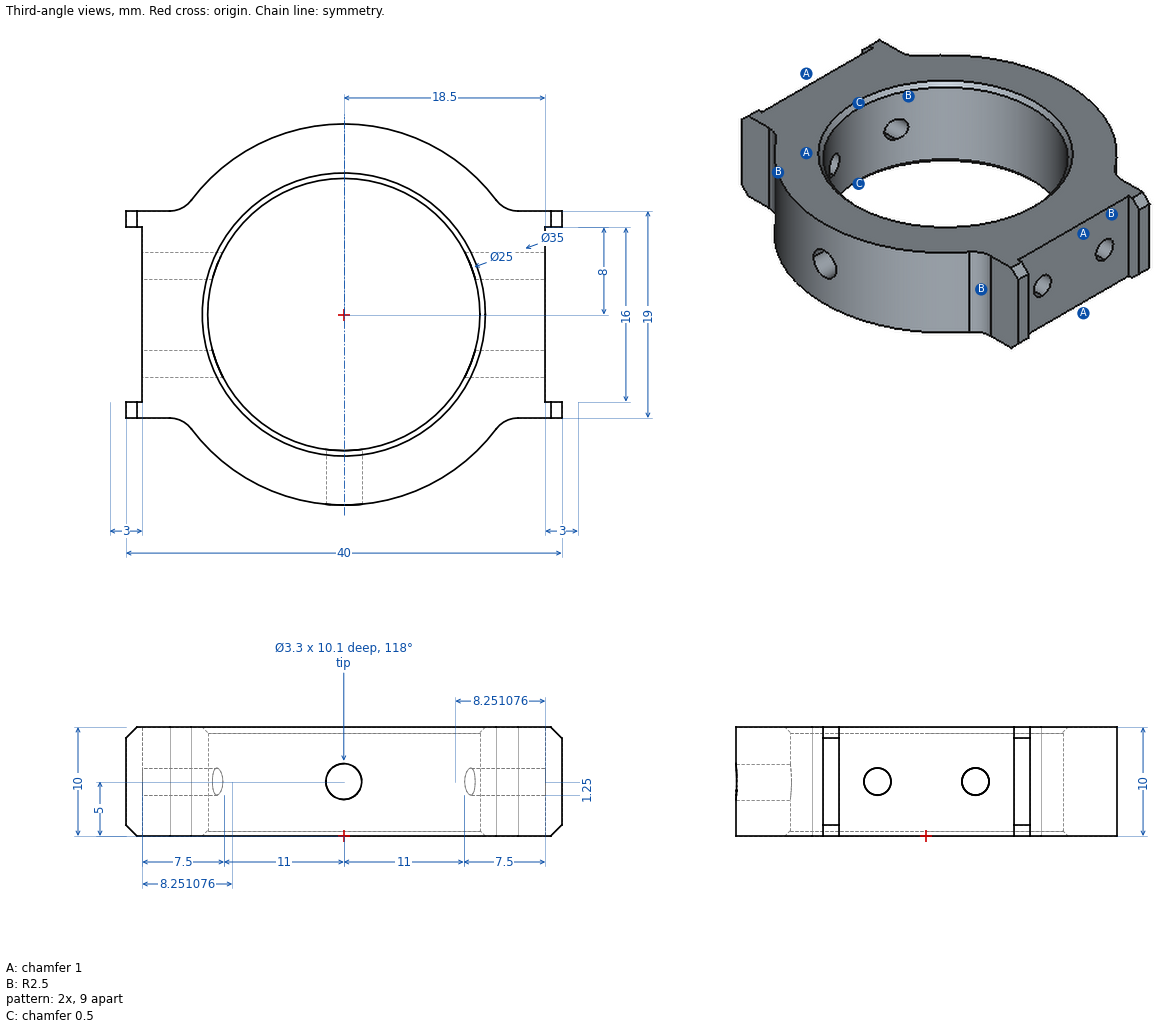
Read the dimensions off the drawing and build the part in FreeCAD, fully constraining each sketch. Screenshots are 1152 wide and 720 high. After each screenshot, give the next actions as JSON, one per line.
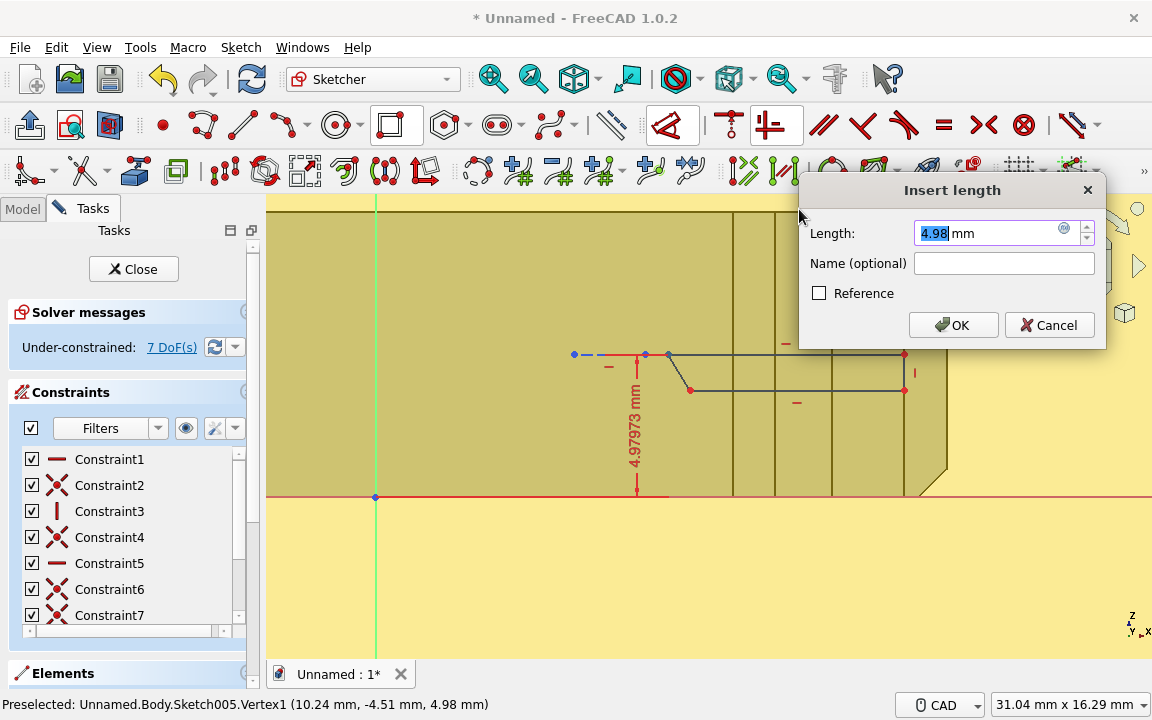
{"action": "type", "text": "5"}
{"action": "key", "text": "Return"}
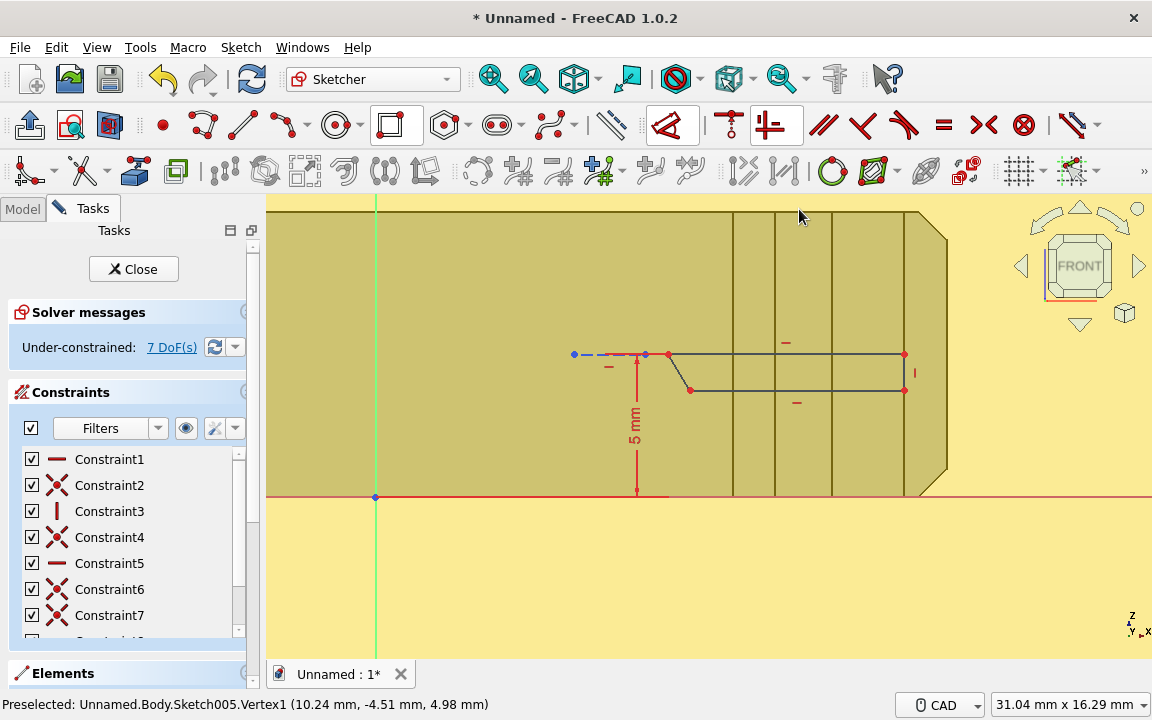
{"action": "left_click", "coordinate": [645, 355]}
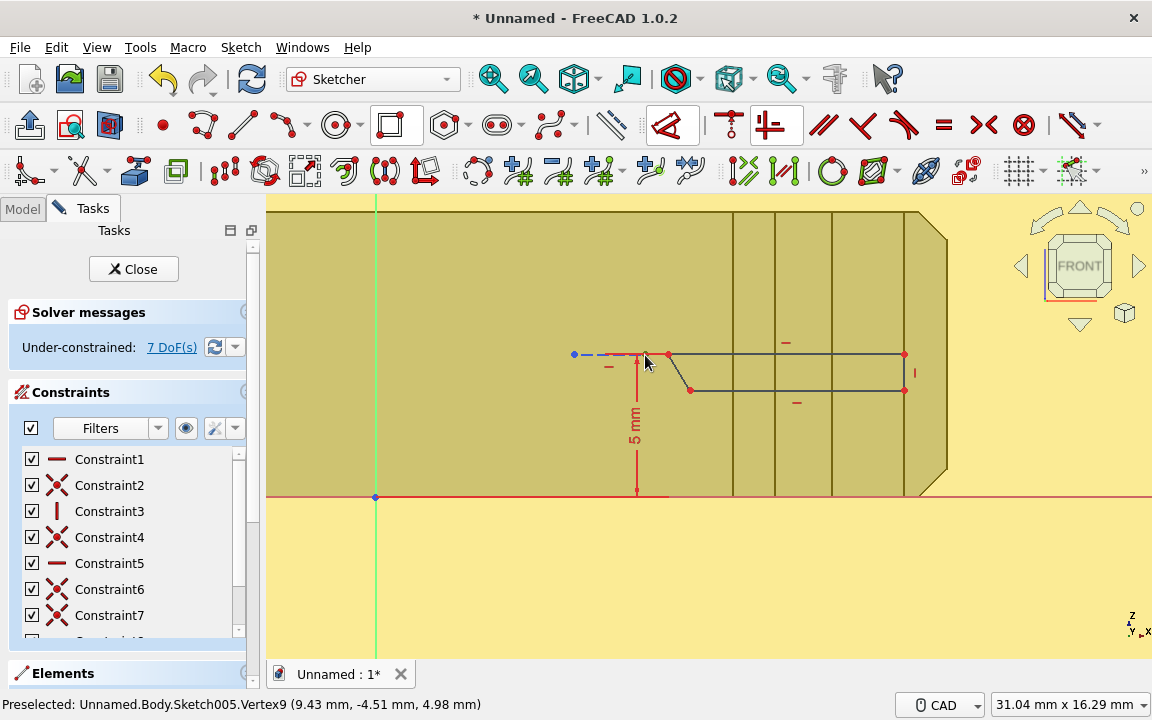
{"action": "key", "text": "i"}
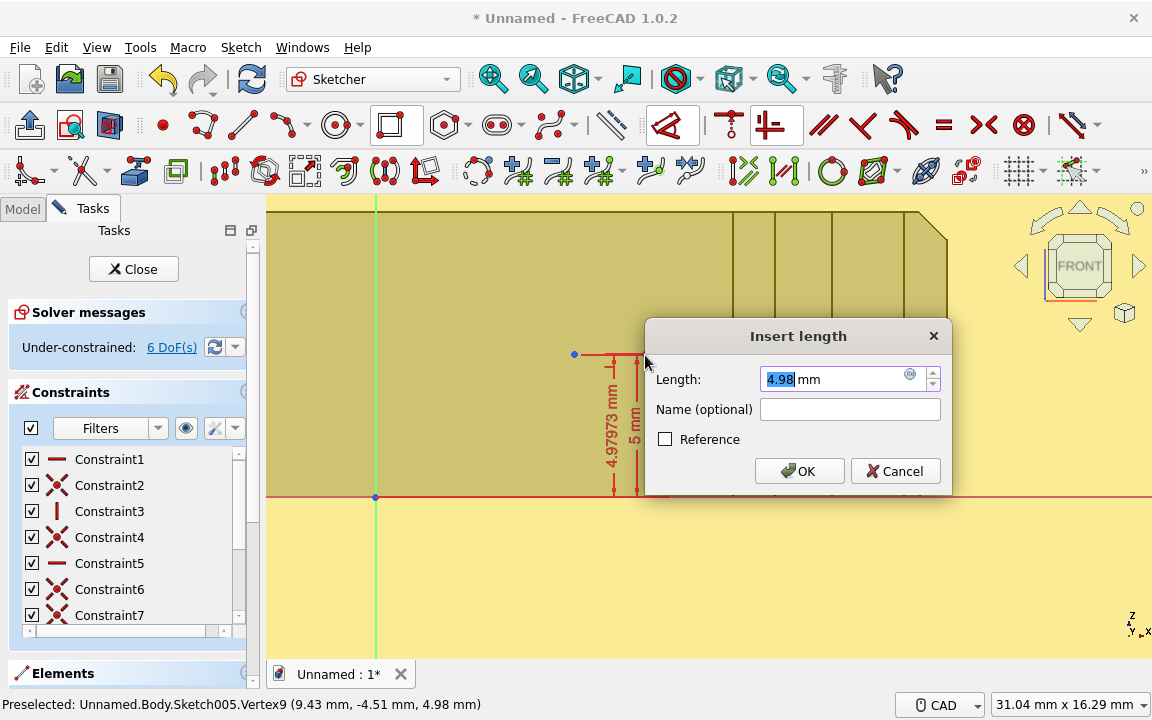
{"action": "type", "text": "5"}
{"action": "key", "text": "Return"}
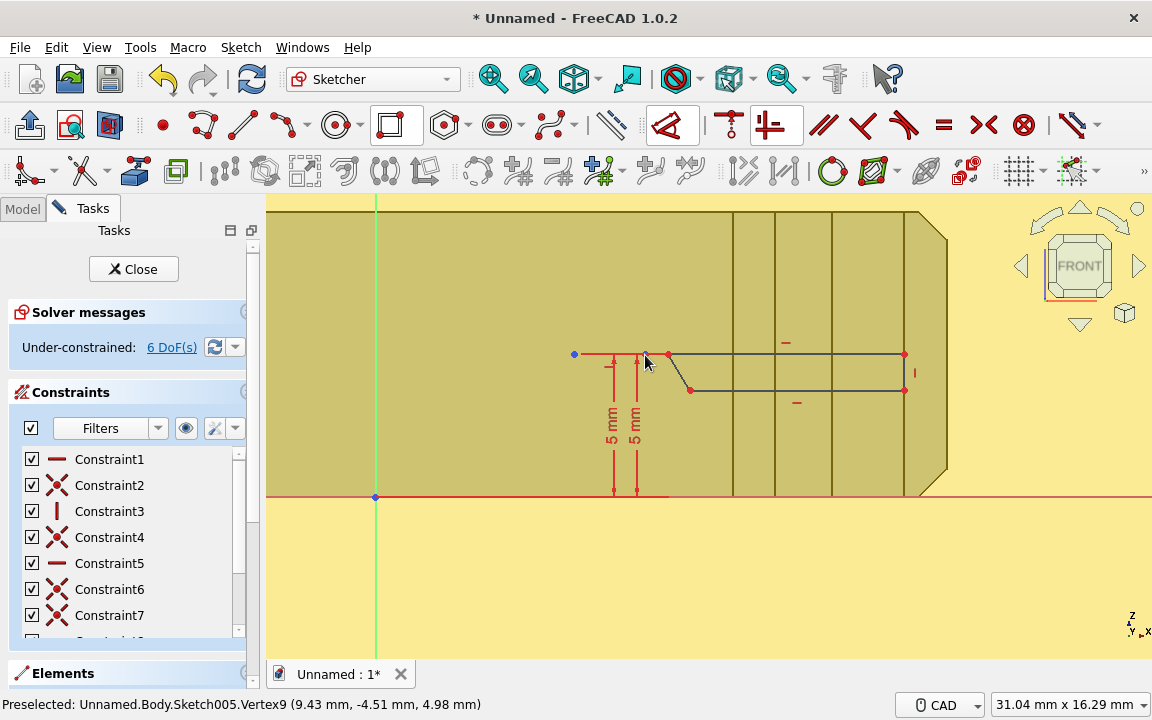
{"action": "left_click", "coordinate": [840, 391]}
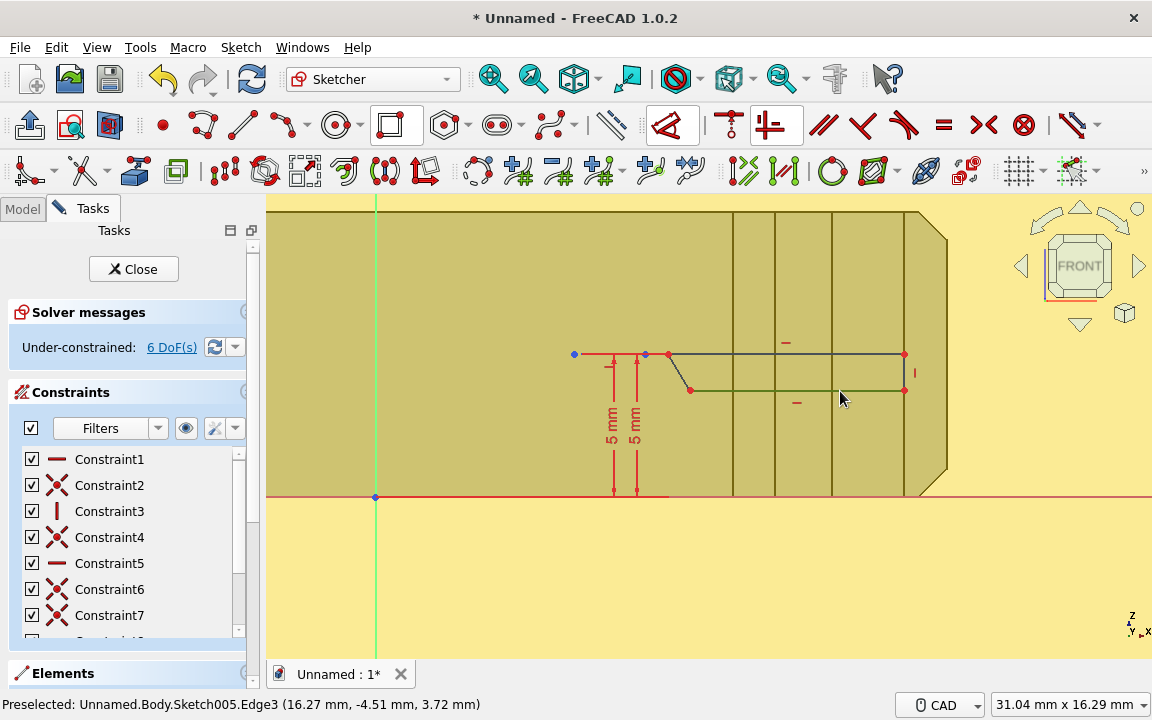
{"action": "left_click", "coordinate": [694, 126]}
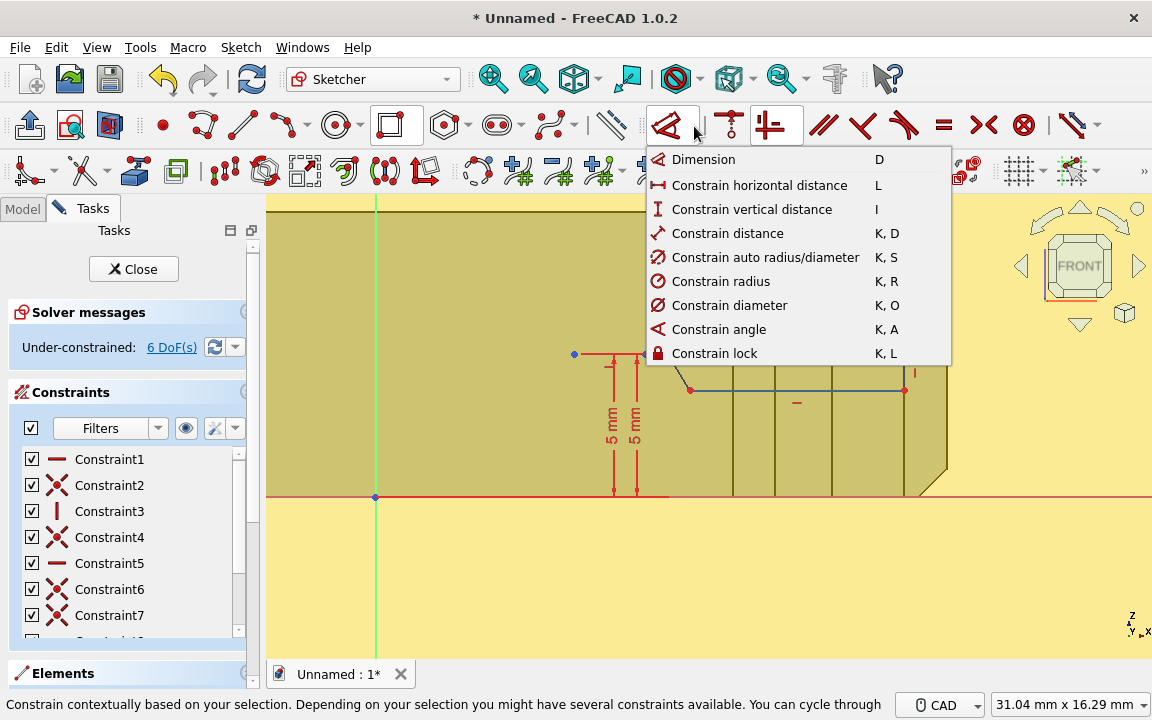
{"action": "left_click", "coordinate": [799, 185]}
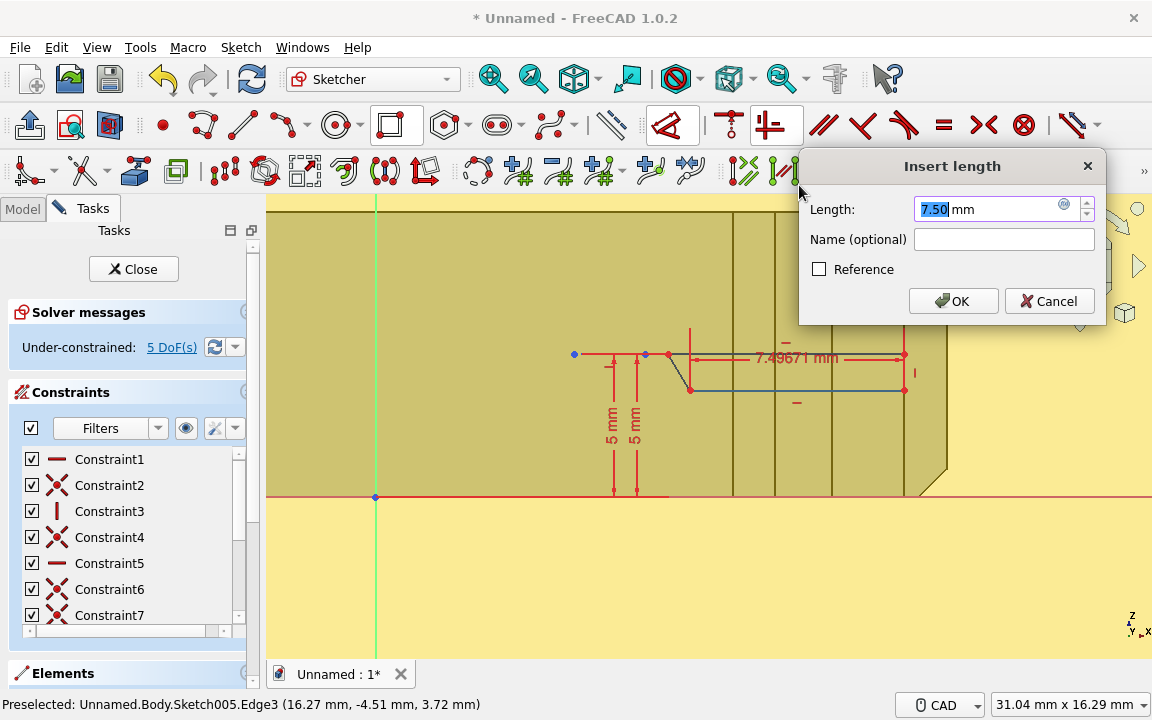
{"action": "type", "text": "7.5"}
{"action": "key", "text": "Return"}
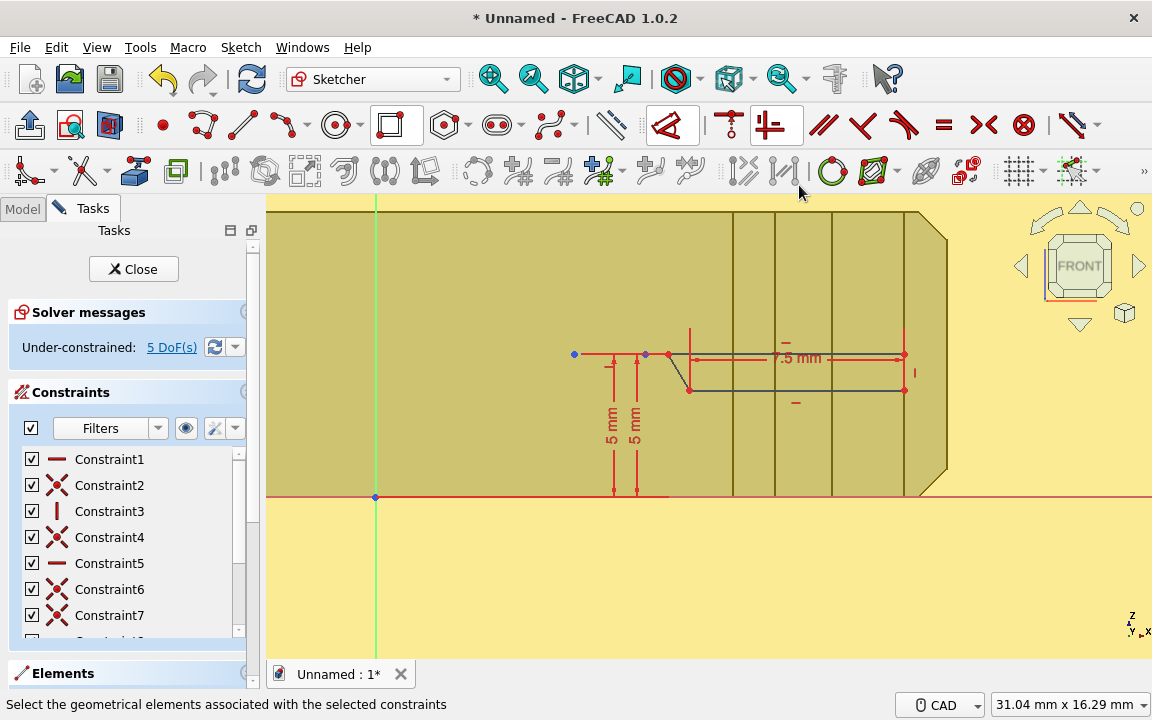
{"action": "left_click", "coordinate": [690, 391]}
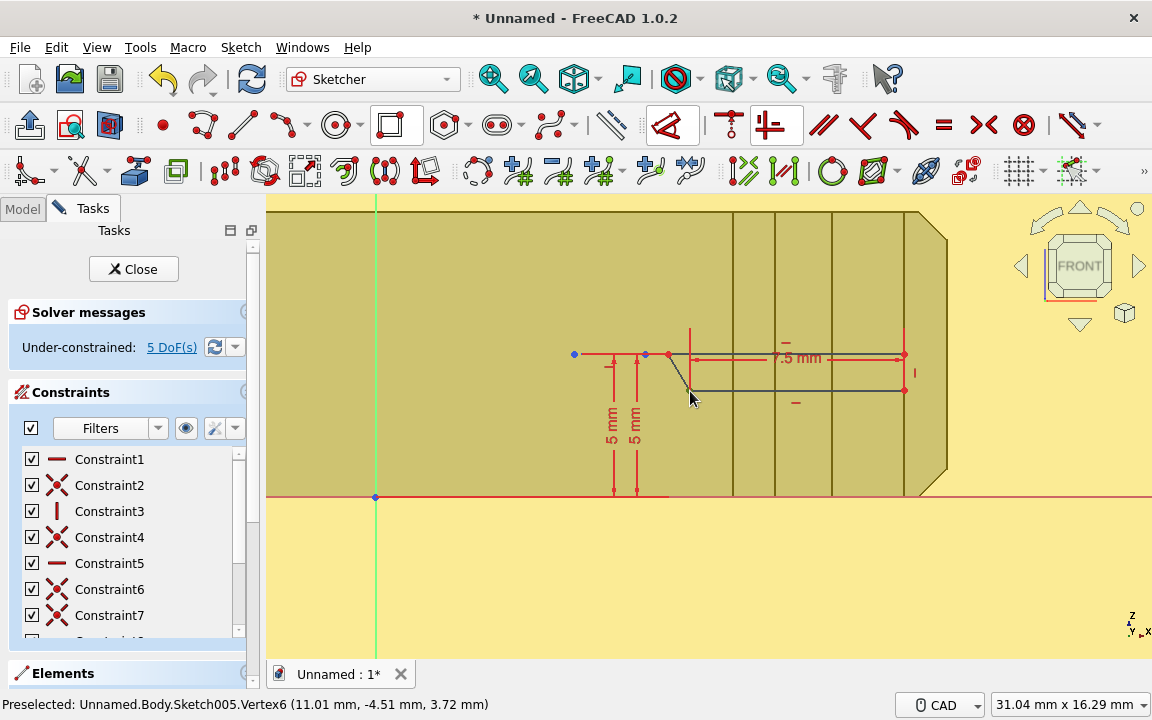
{"action": "left_click", "coordinate": [694, 126]}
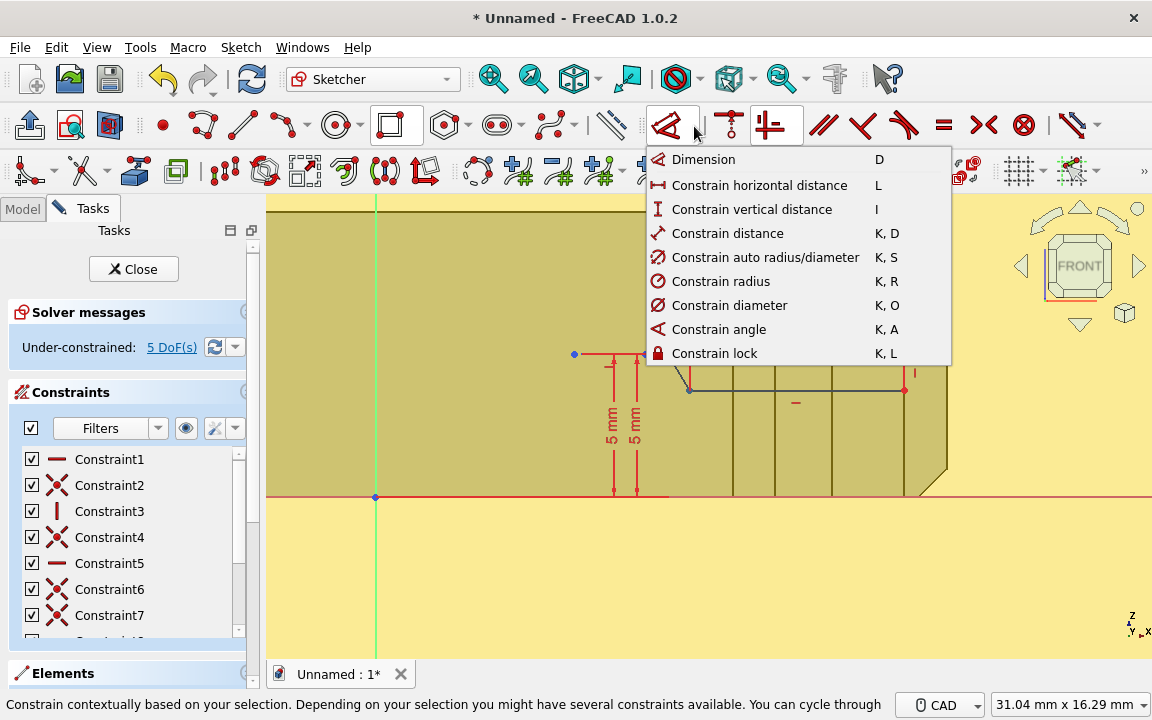
{"action": "left_click", "coordinate": [799, 185]}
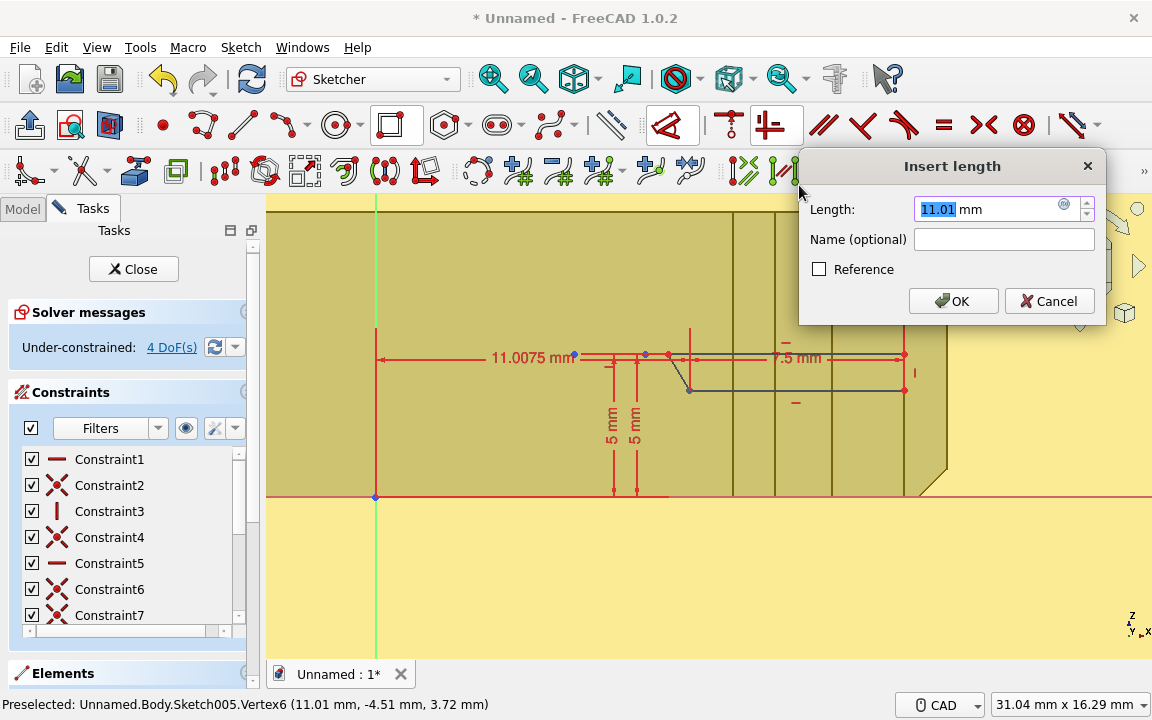
{"action": "type", "text": "11"}
{"action": "key", "text": "Return"}